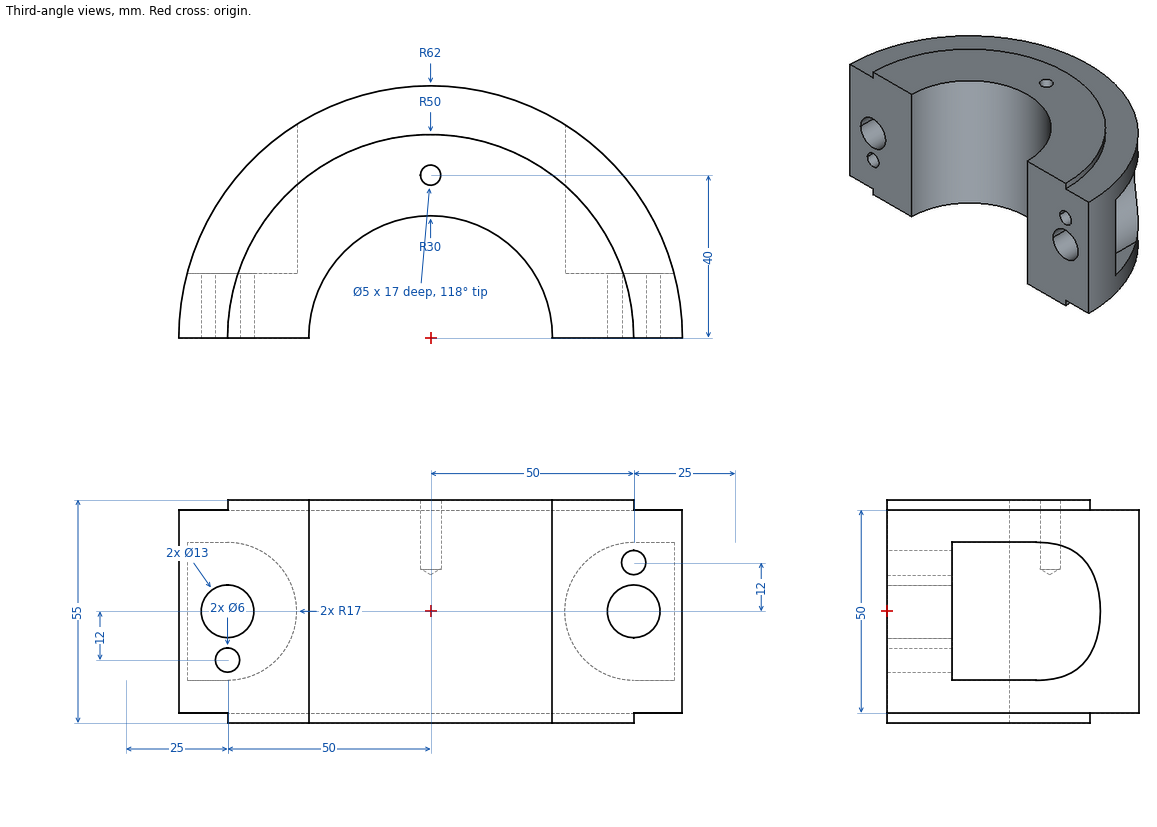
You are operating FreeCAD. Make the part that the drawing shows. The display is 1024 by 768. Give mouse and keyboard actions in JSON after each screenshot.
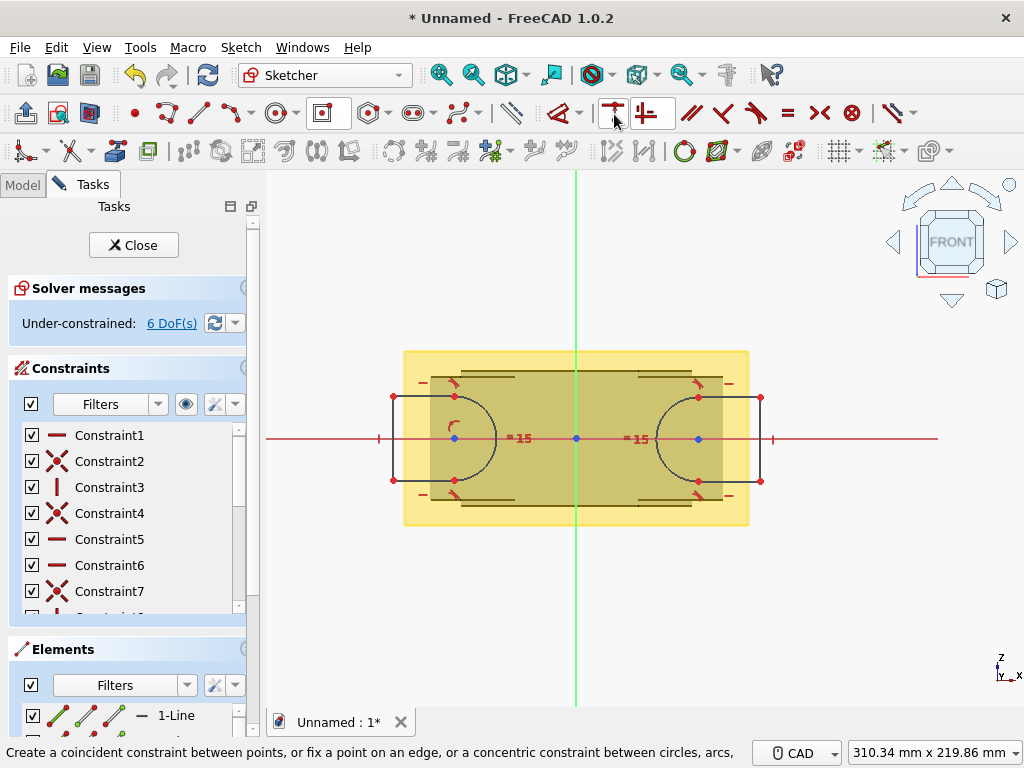
{"action": "left_click", "coordinate": [699, 439]}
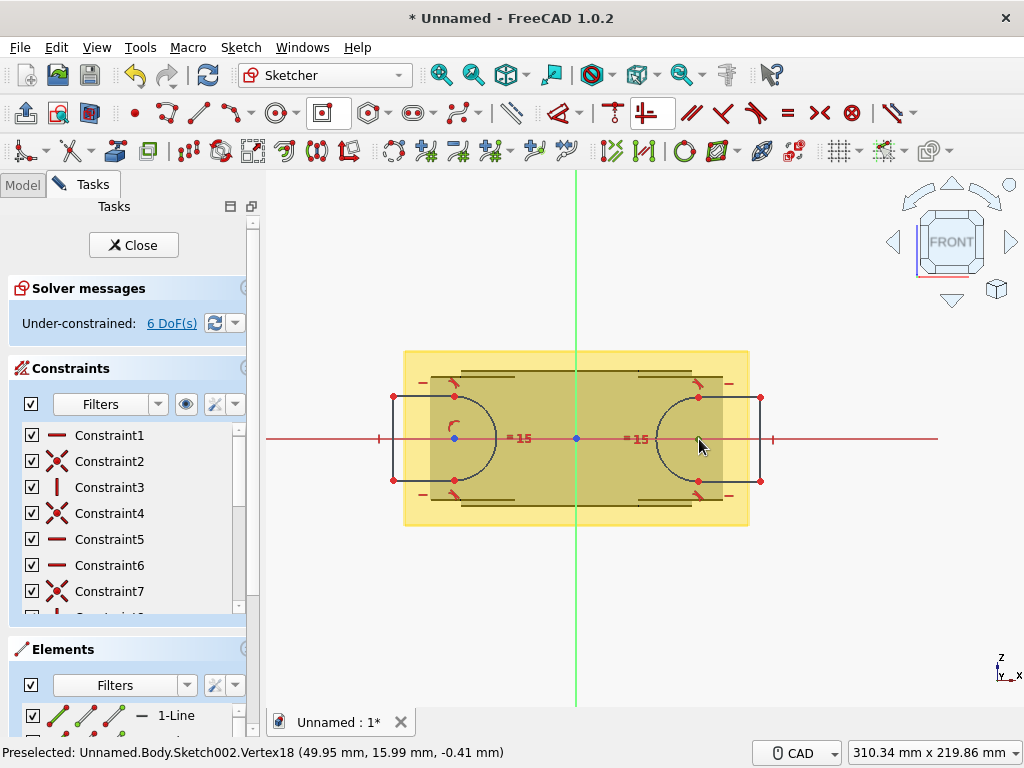
{"action": "left_click", "coordinate": [334, 439]}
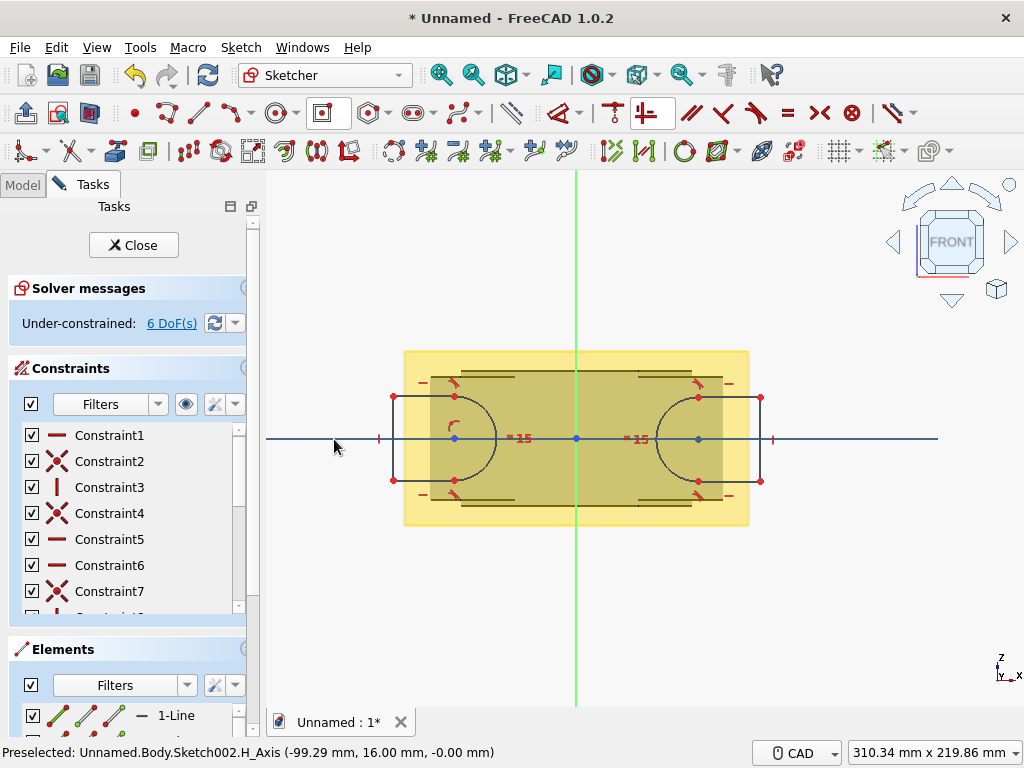
{"action": "key", "text": "c"}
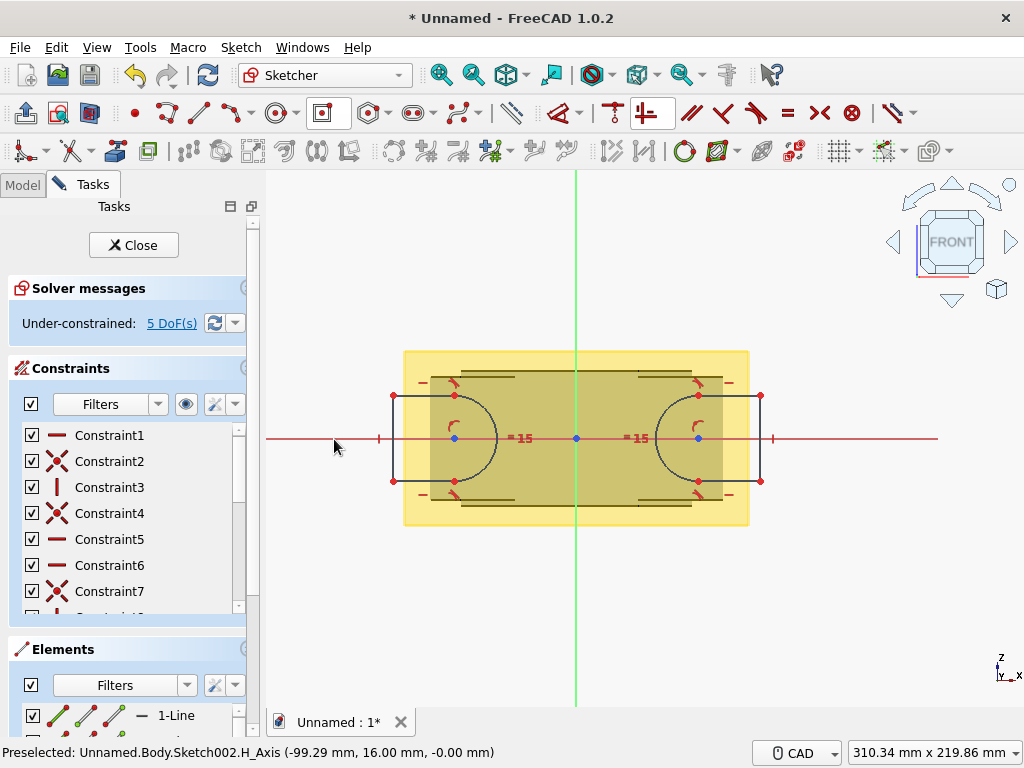
{"action": "left_click", "coordinate": [558, 114]}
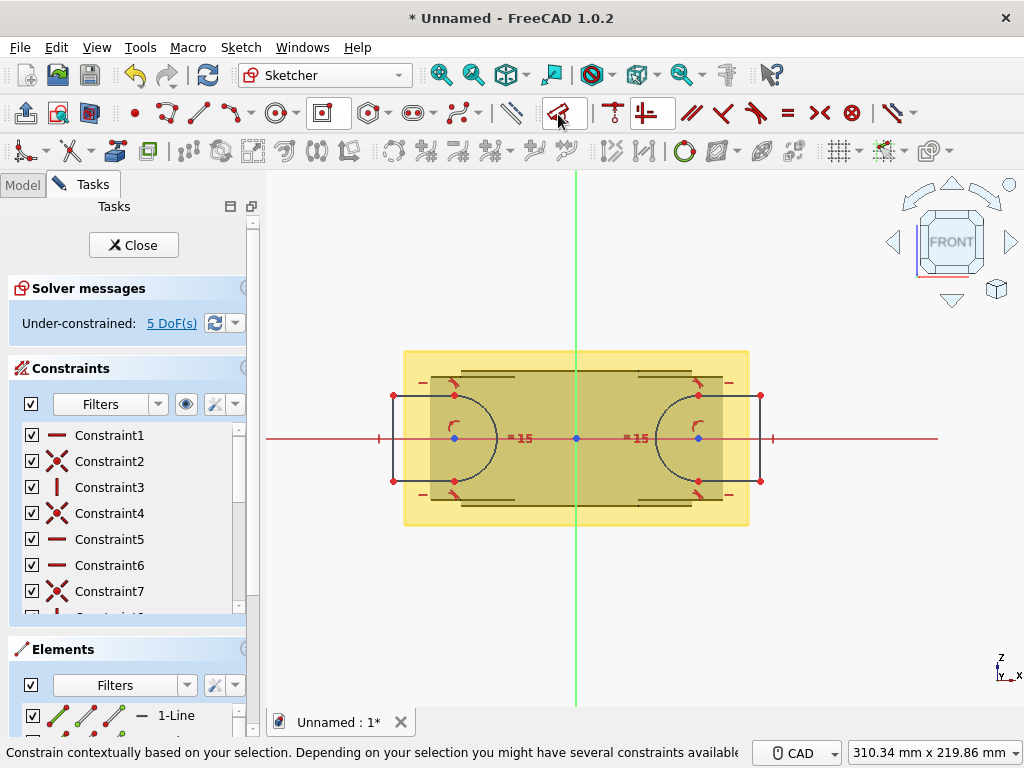
{"action": "left_click", "coordinate": [489, 464]}
{"action": "left_click", "coordinate": [515, 483]}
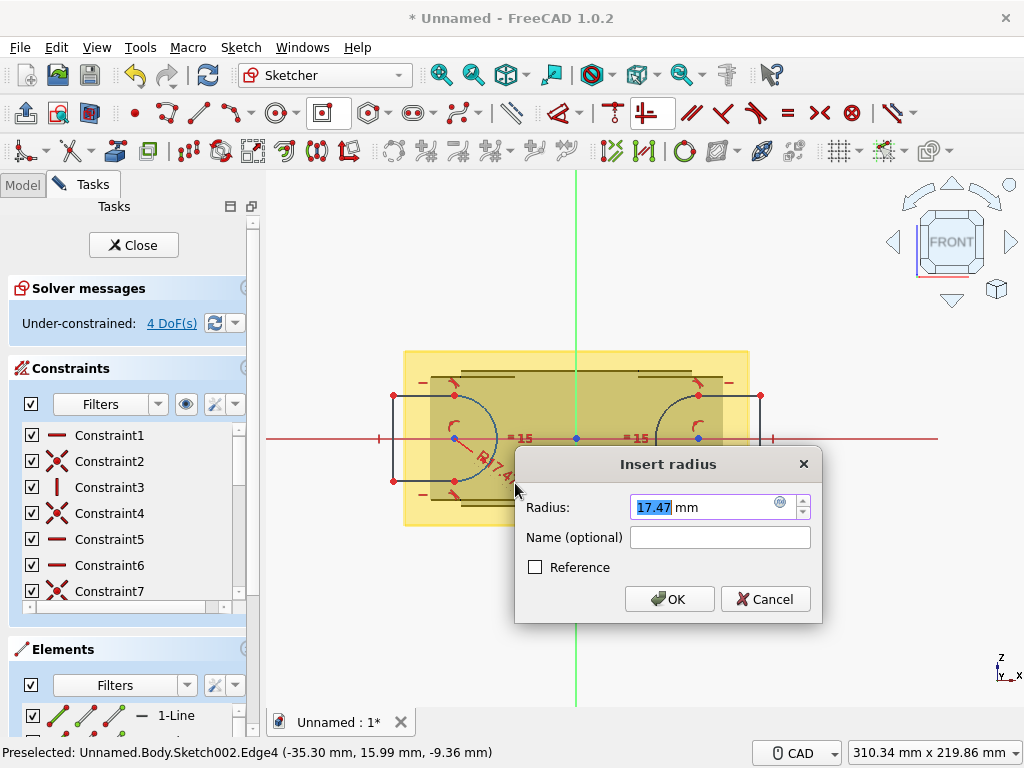
{"action": "type", "text": "17"}
{"action": "key", "text": "Return"}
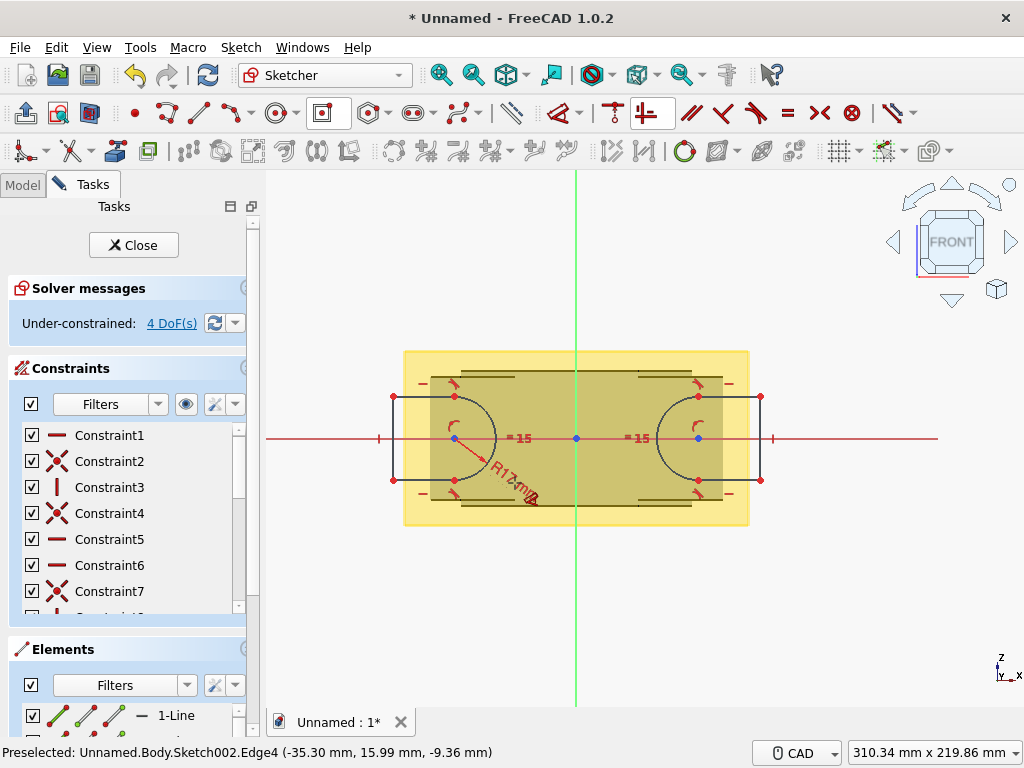
{"action": "left_click", "coordinate": [436, 480]}
{"action": "left_click", "coordinate": [424, 514]}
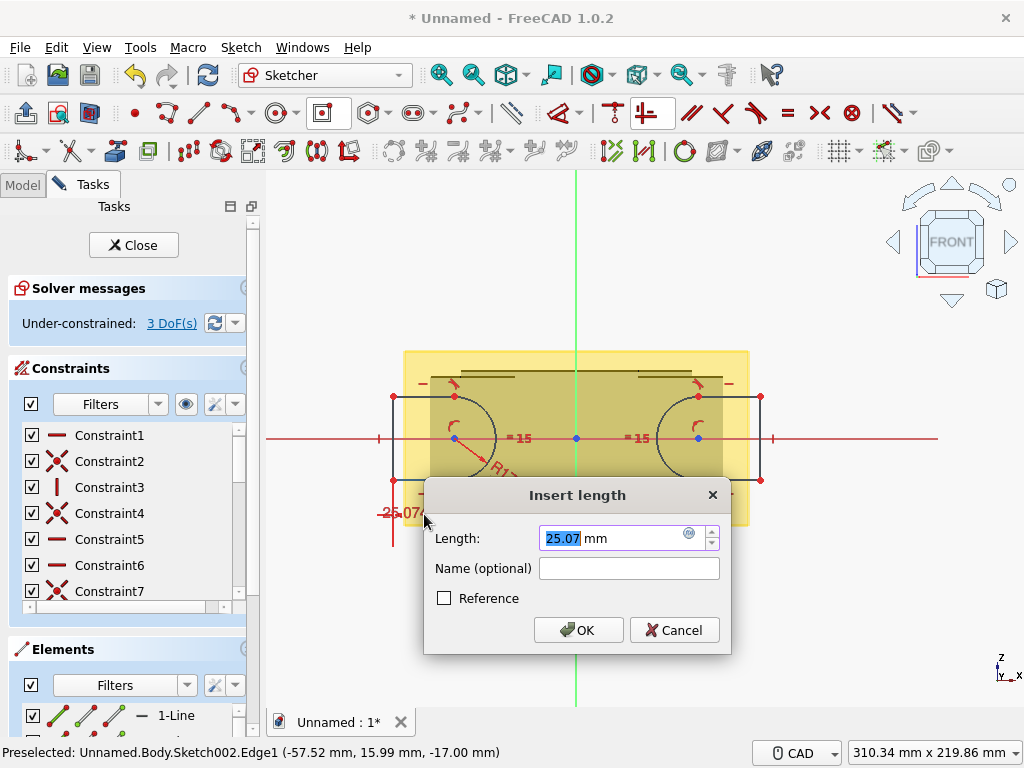
{"action": "type", "text": "25"}
{"action": "key", "text": "Return"}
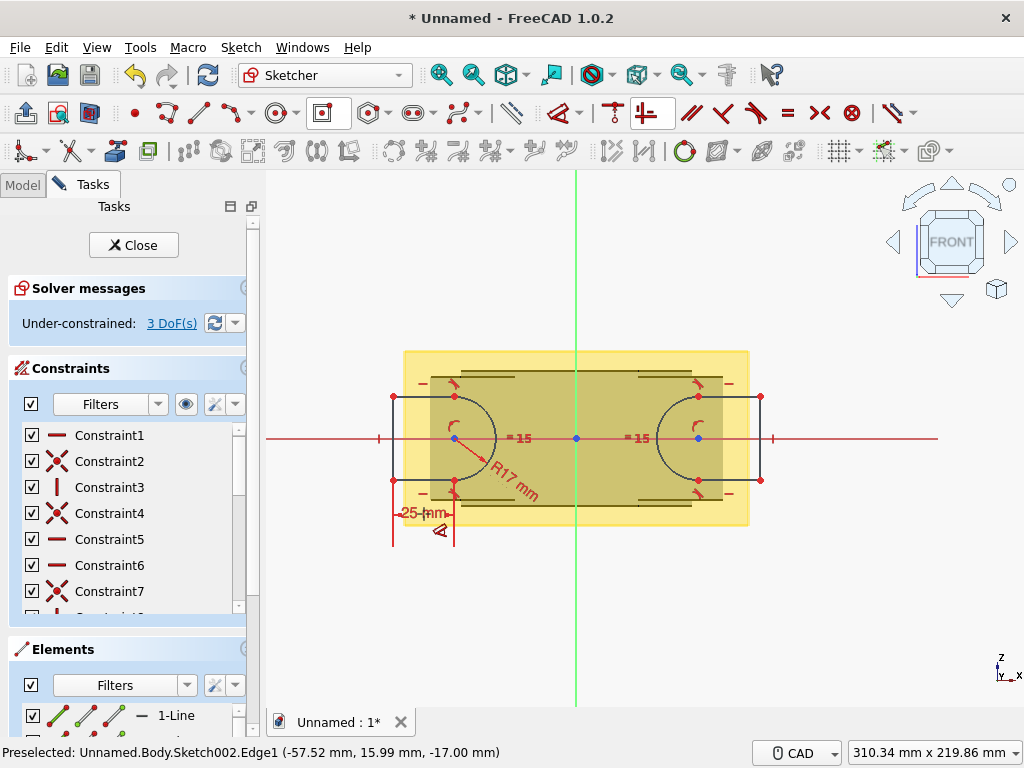
{"action": "left_click", "coordinate": [717, 397]}
{"action": "left_click", "coordinate": [729, 363]}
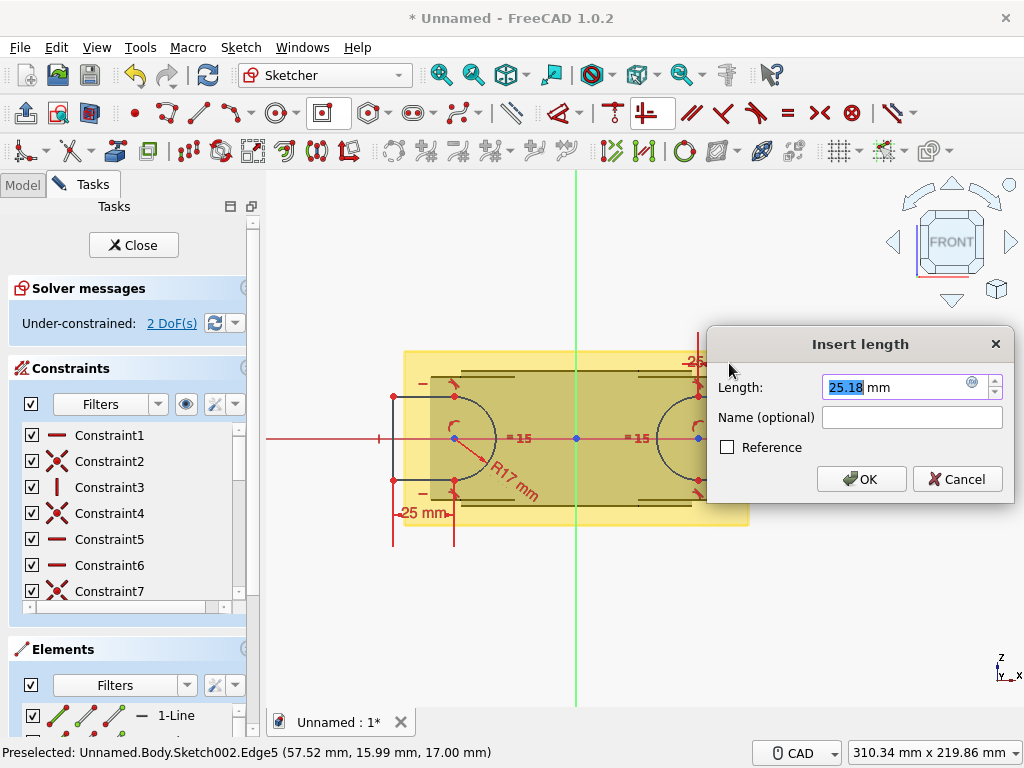
{"action": "type", "text": "25"}
{"action": "key", "text": "Return"}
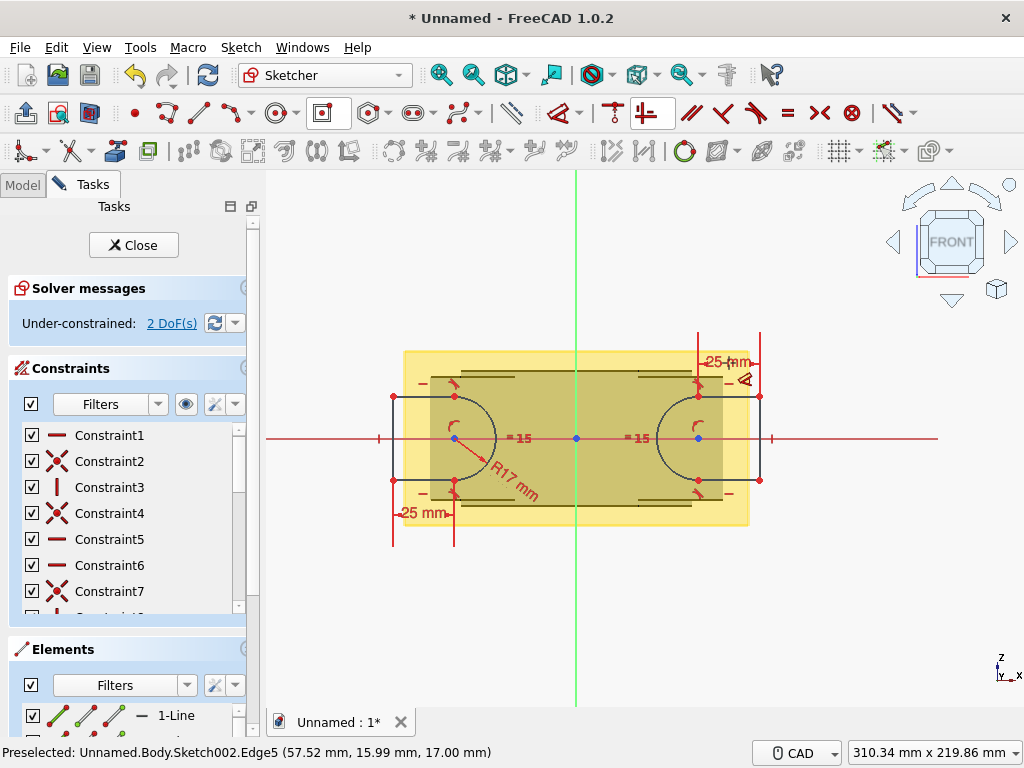
{"action": "left_click", "coordinate": [454, 480]}
{"action": "left_click", "coordinate": [515, 514]}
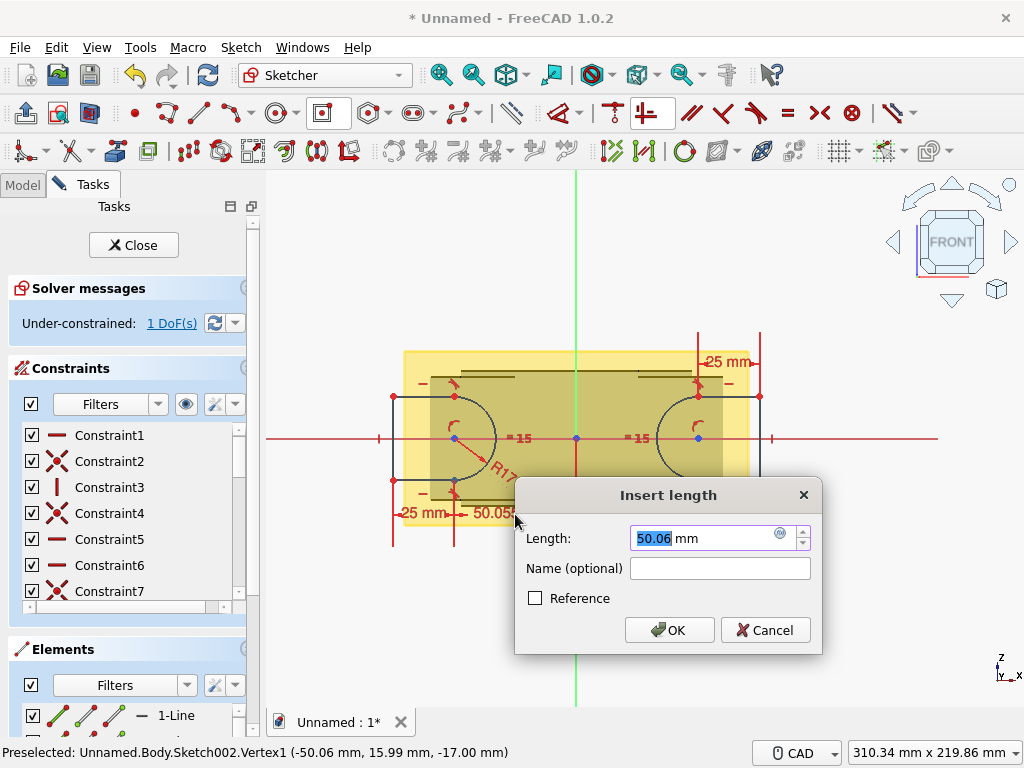
{"action": "type", "text": "50"}
{"action": "key", "text": "Return"}